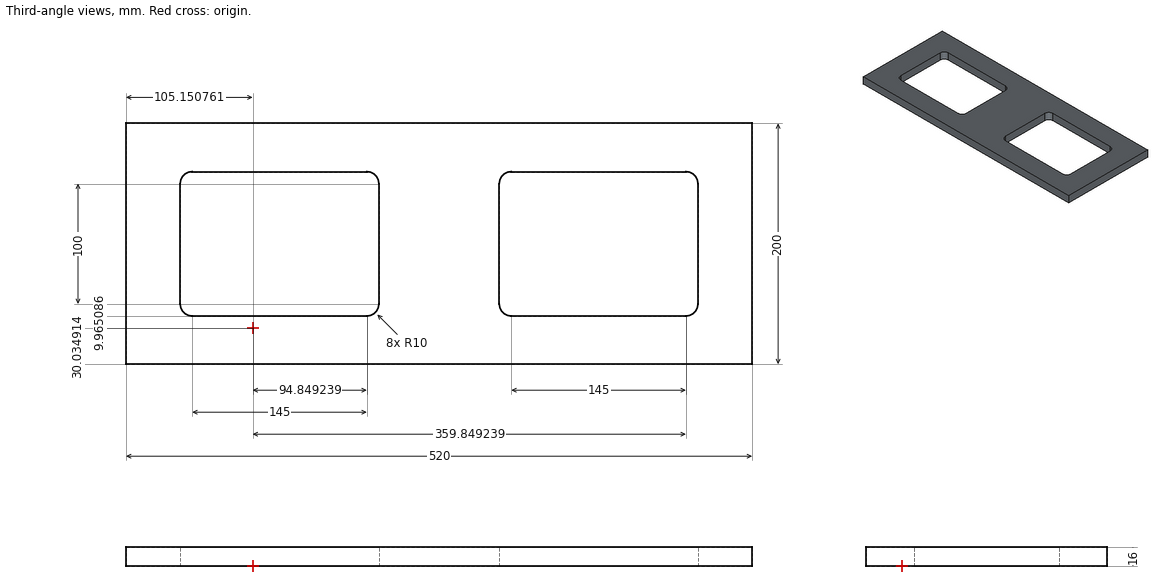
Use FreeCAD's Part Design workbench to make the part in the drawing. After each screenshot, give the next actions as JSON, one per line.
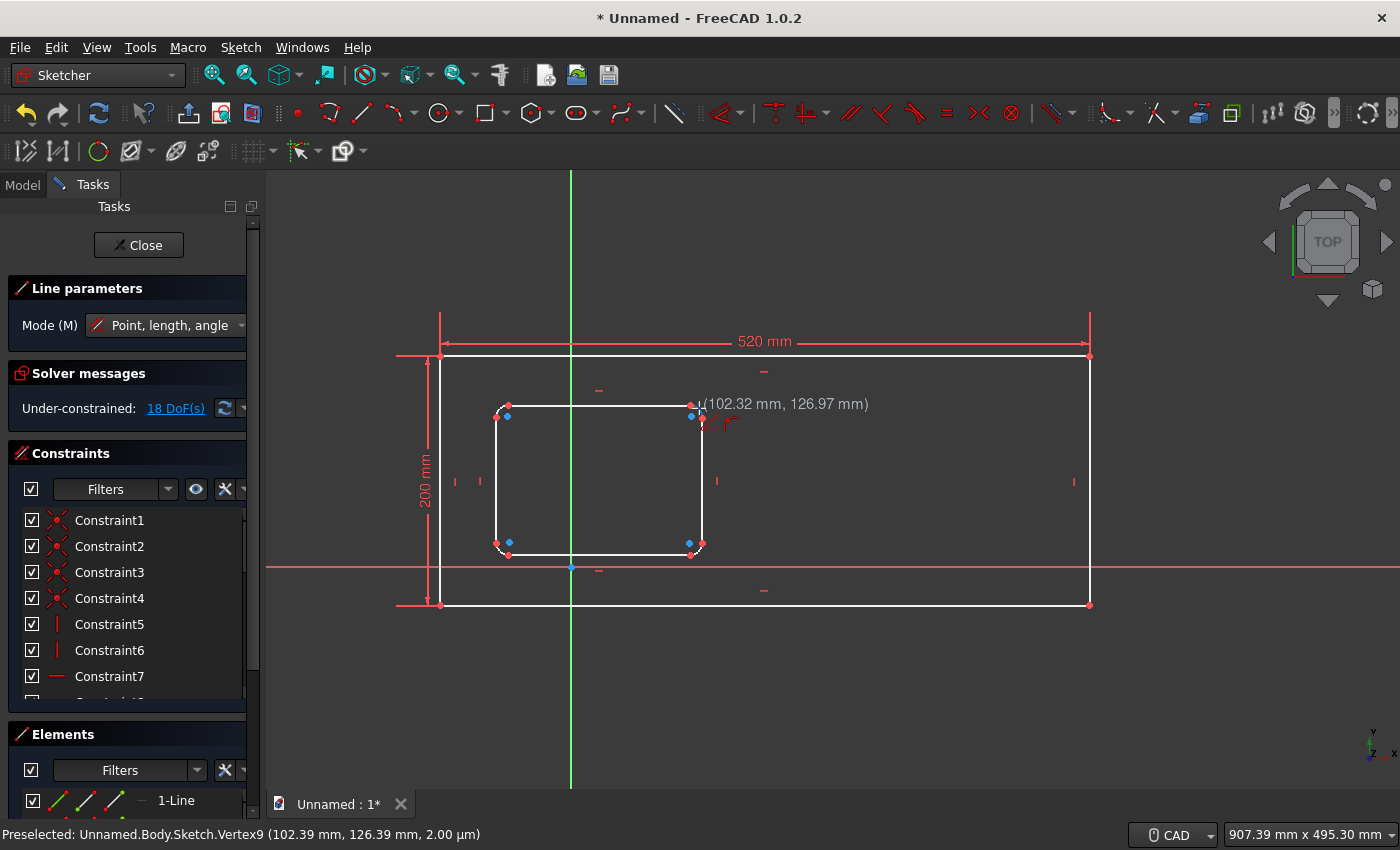
{"action": "scroll", "coordinate": [1021, 555], "scroll_direction": "up", "scroll_amount": 2}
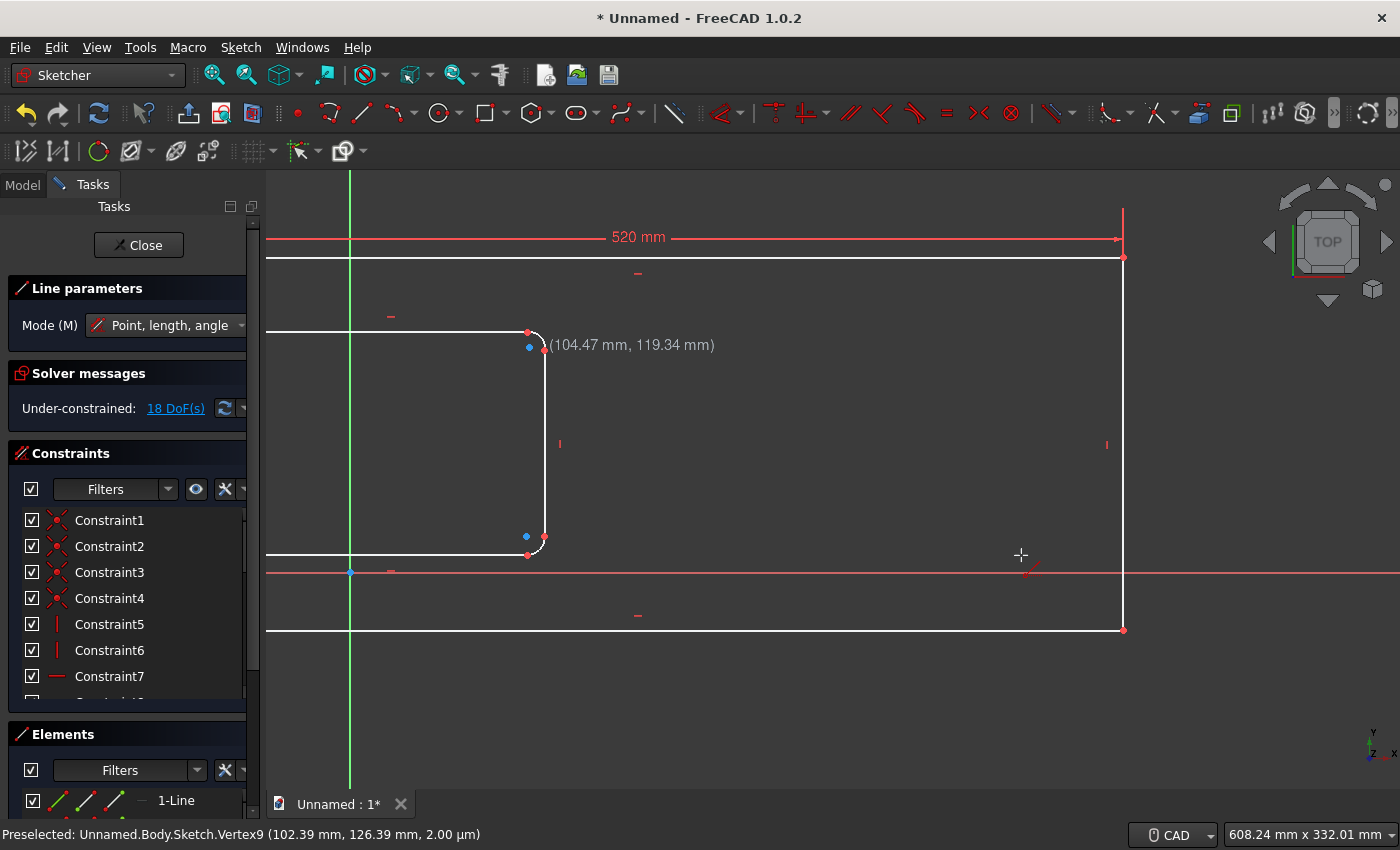
{"action": "left_click", "coordinate": [1021, 554]}
{"action": "left_click", "coordinate": [751, 554]}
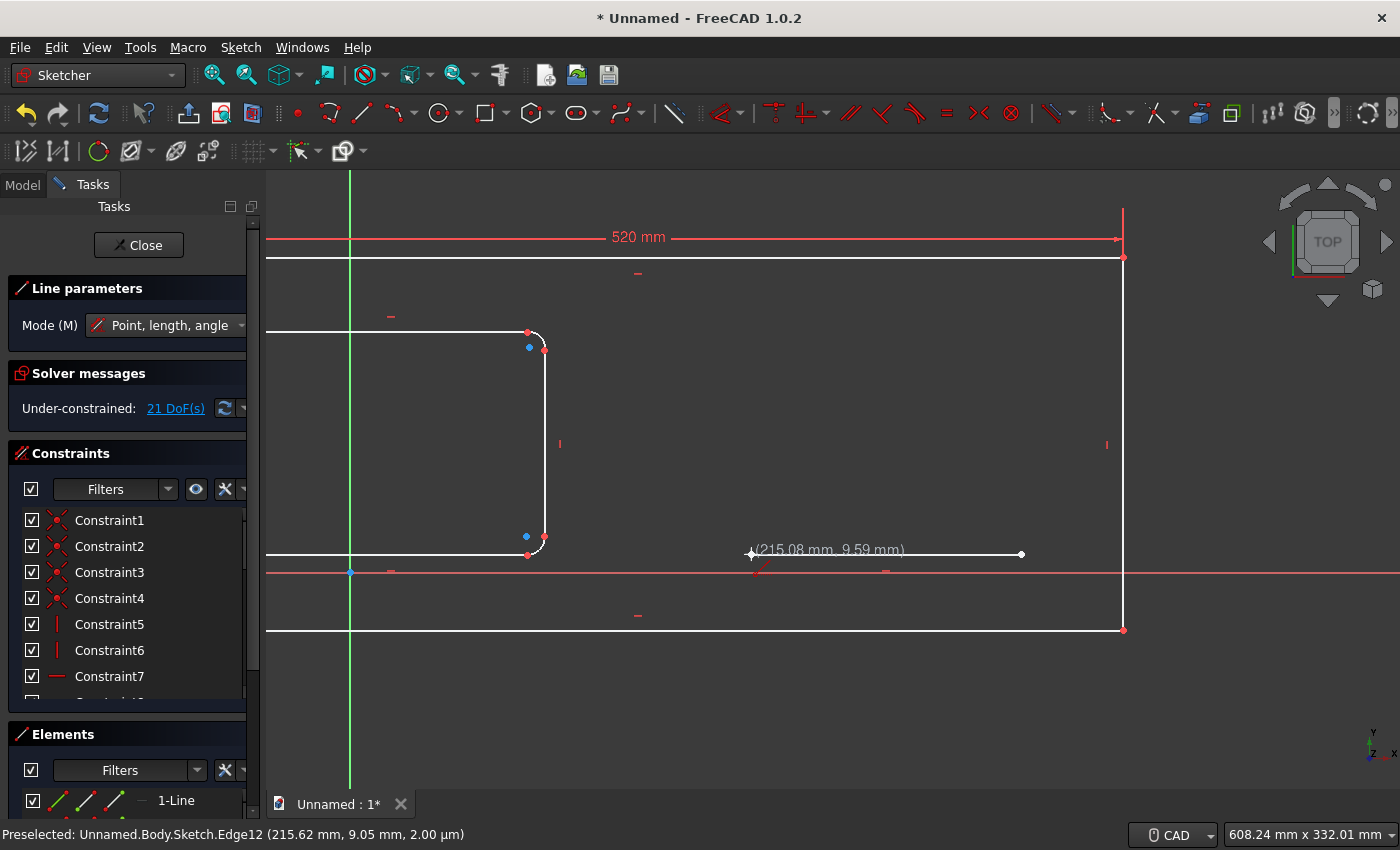
{"action": "left_click", "coordinate": [732, 536]}
{"action": "left_click", "coordinate": [732, 349]}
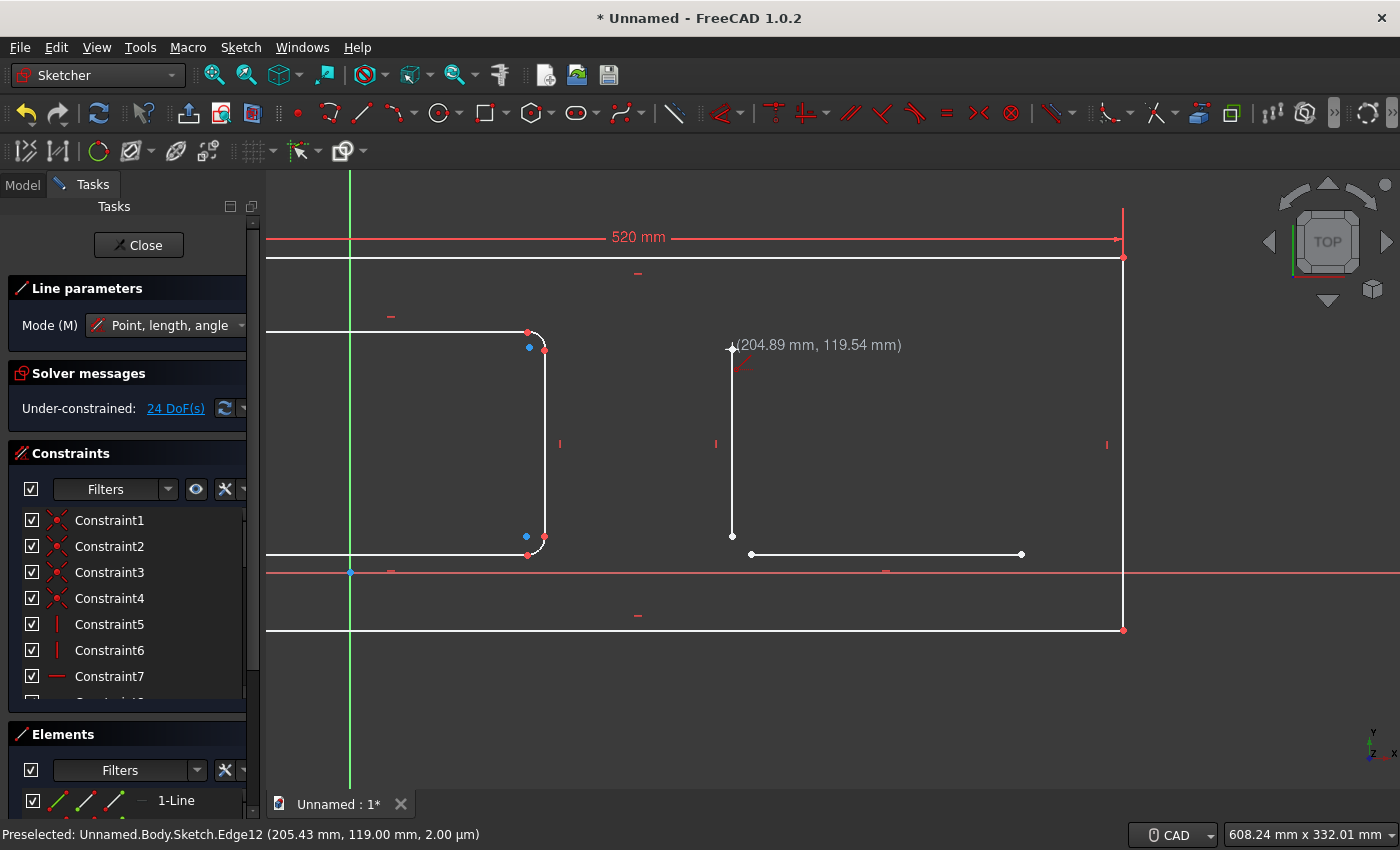
{"action": "left_click", "coordinate": [751, 331]}
{"action": "left_click", "coordinate": [1021, 331]}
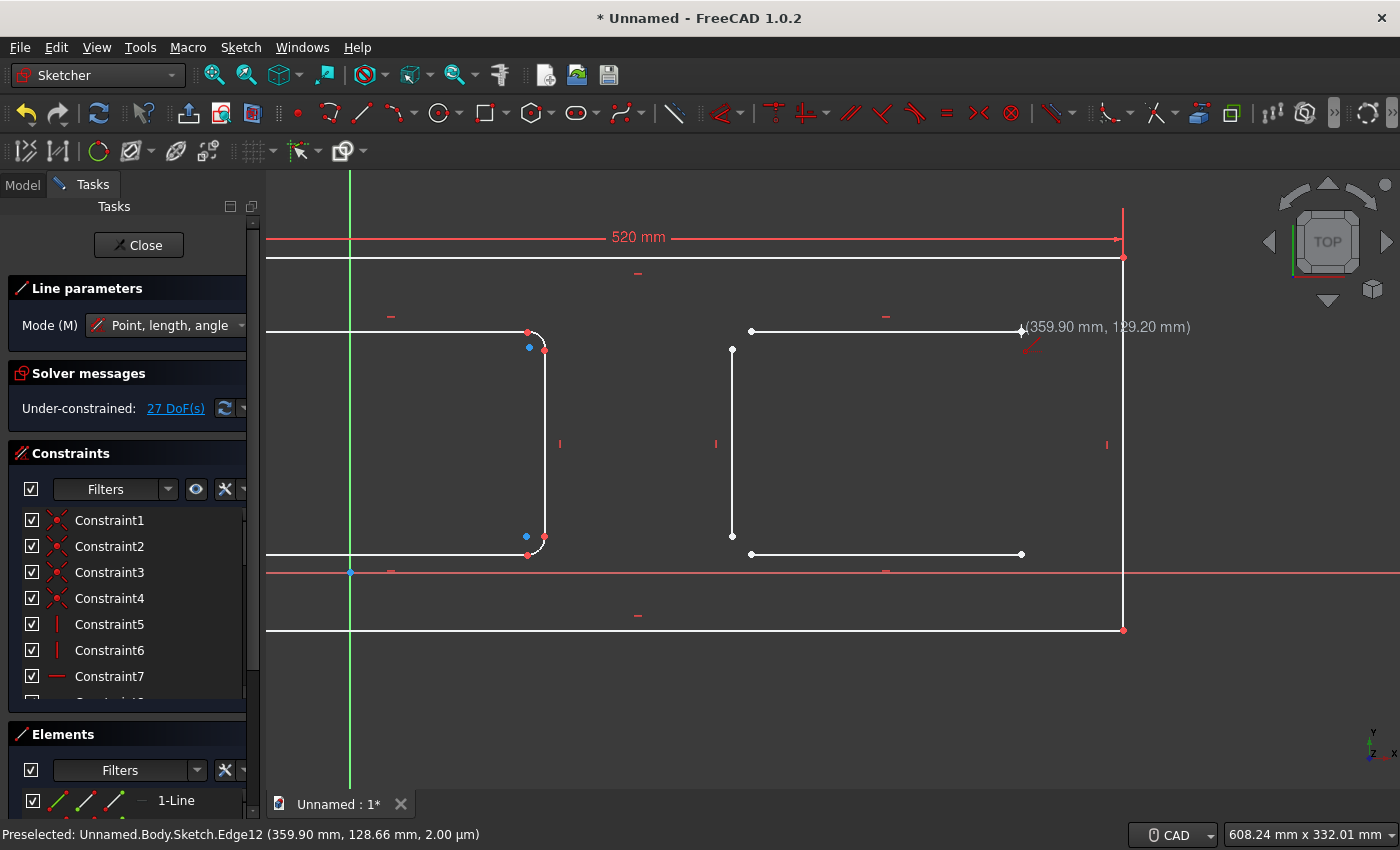
{"action": "left_click", "coordinate": [1040, 349]}
{"action": "left_click", "coordinate": [1040, 536]}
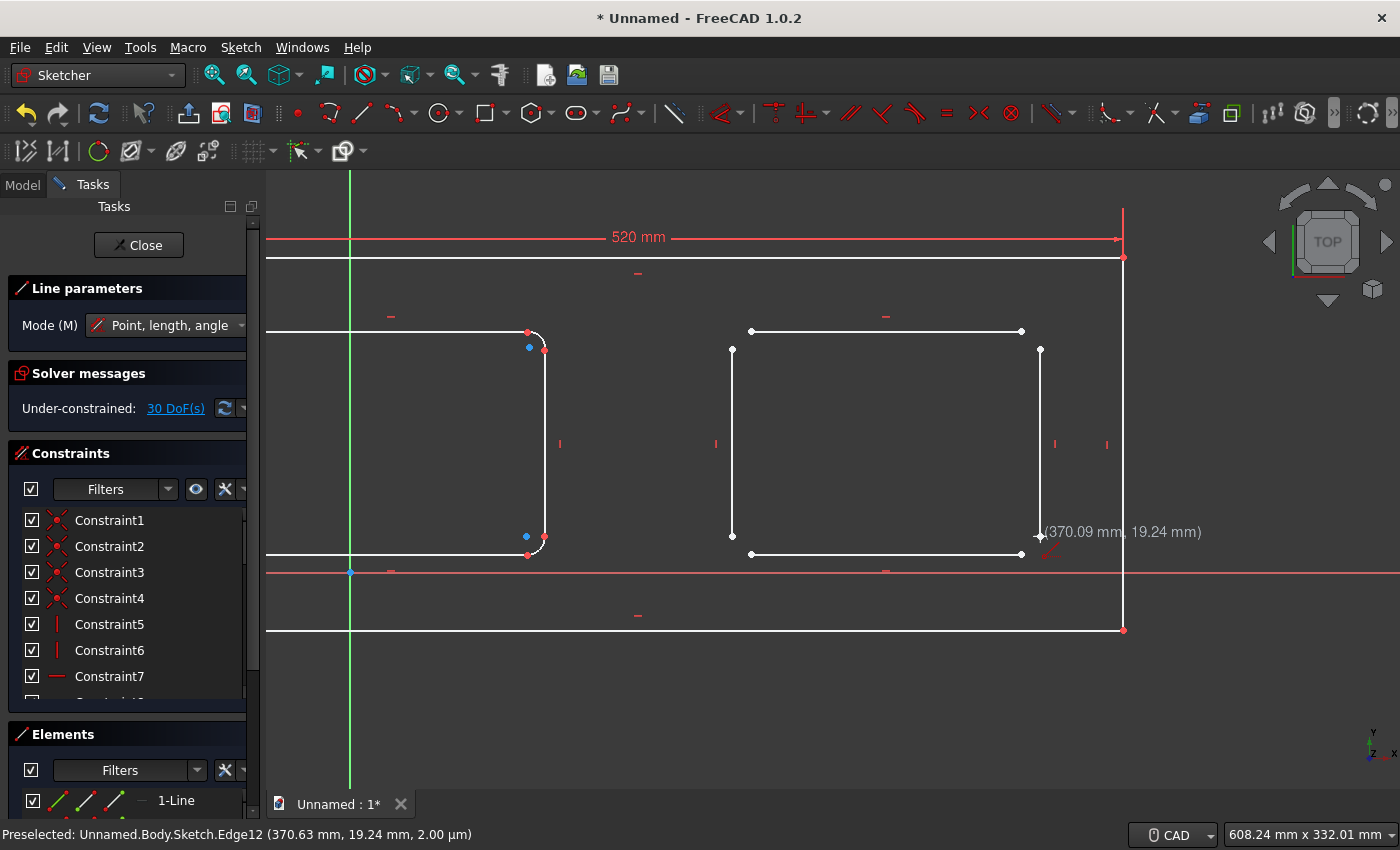
{"action": "left_click", "coordinate": [394, 114]}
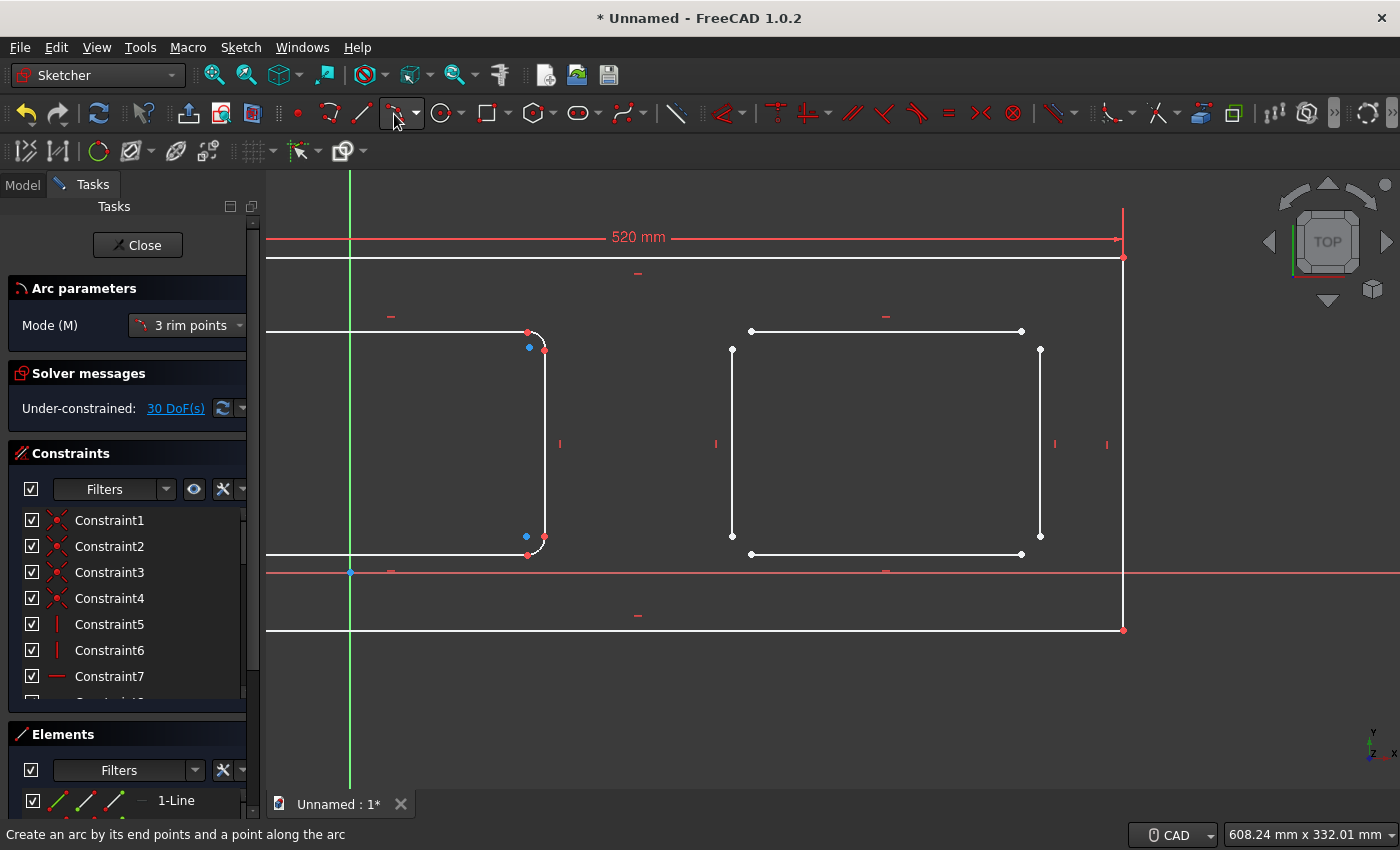
{"action": "left_click", "coordinate": [751, 555]}
{"action": "left_click", "coordinate": [732, 537]}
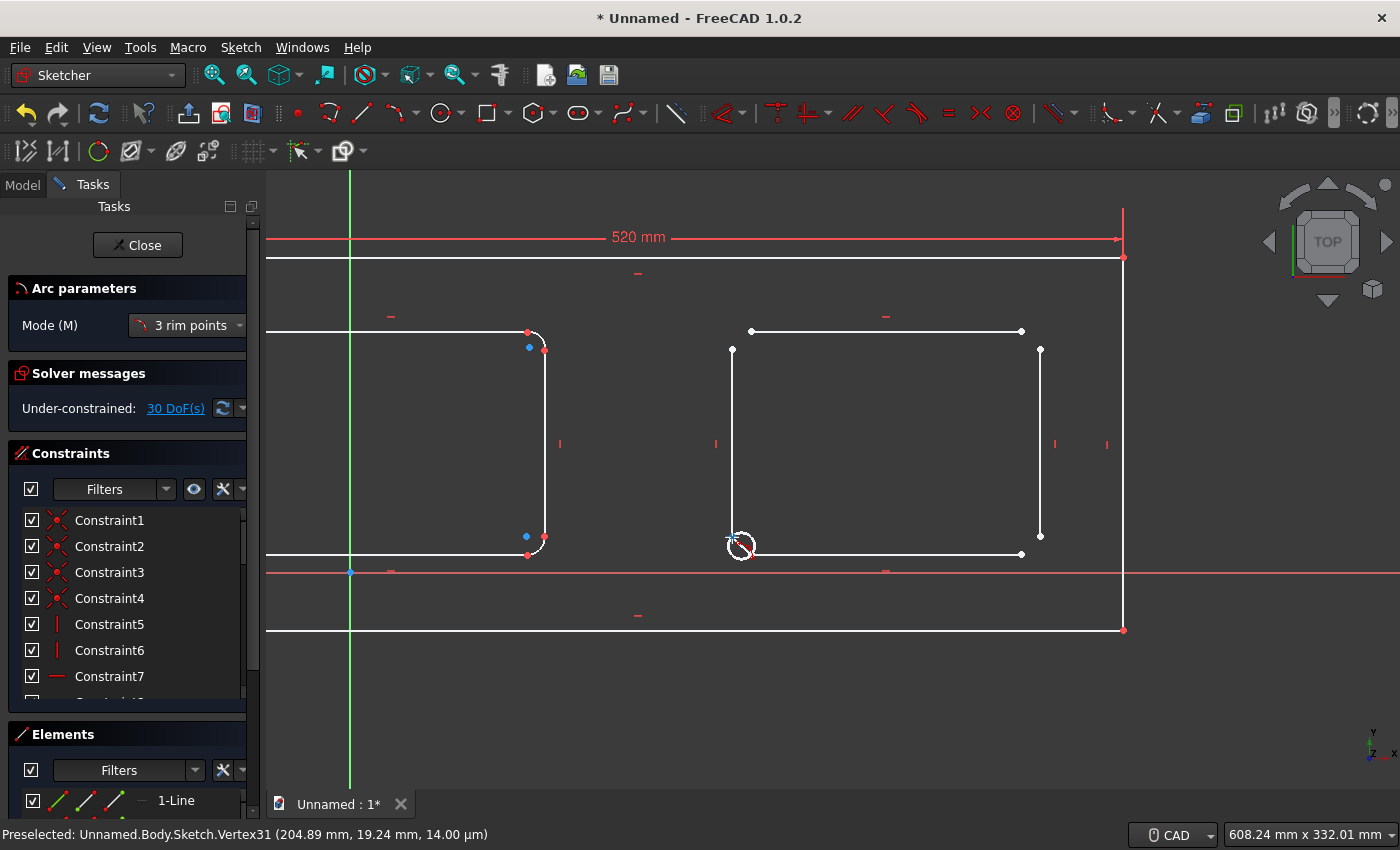
{"action": "scroll", "coordinate": [737, 549], "scroll_direction": "up", "scroll_amount": 6}